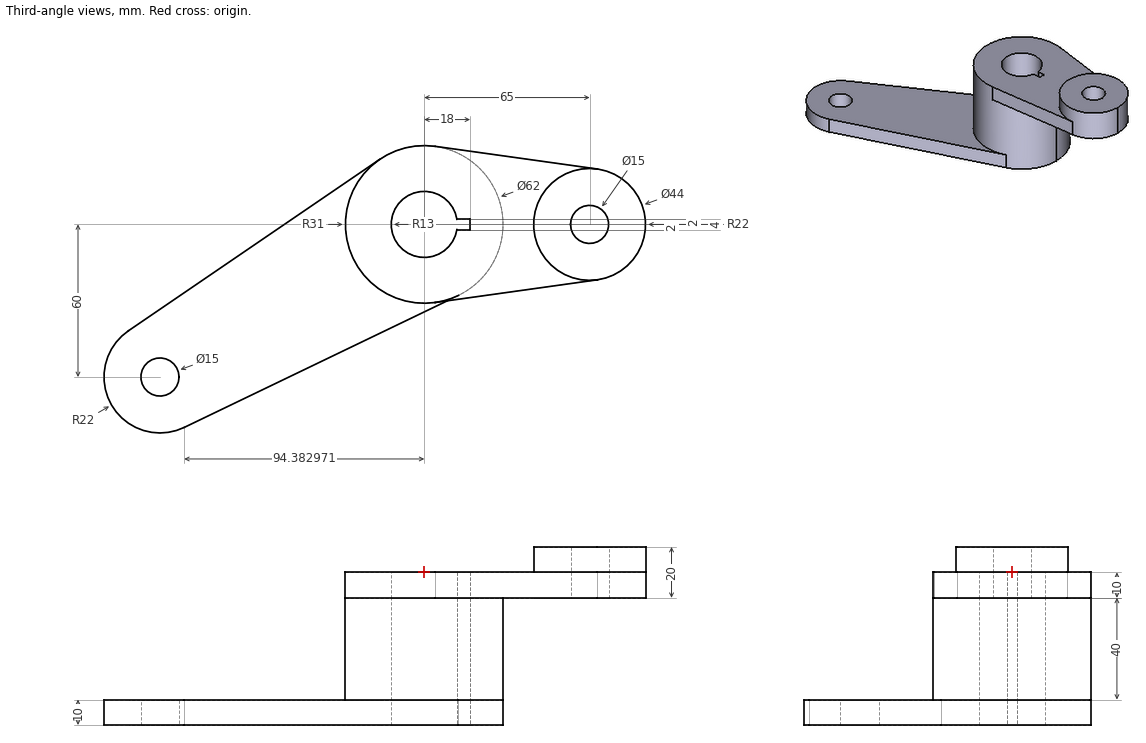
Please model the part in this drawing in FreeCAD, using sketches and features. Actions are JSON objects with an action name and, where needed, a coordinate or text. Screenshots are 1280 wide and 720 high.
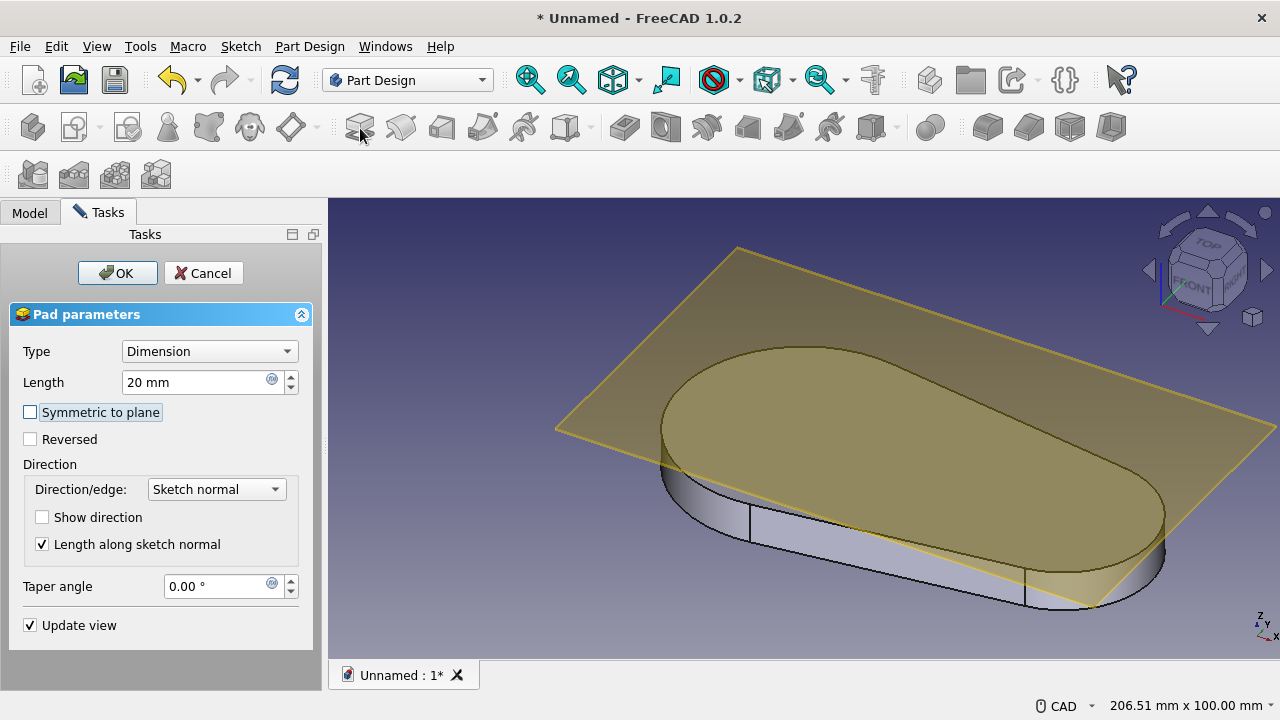
{"action": "left_click", "coordinate": [31, 439]}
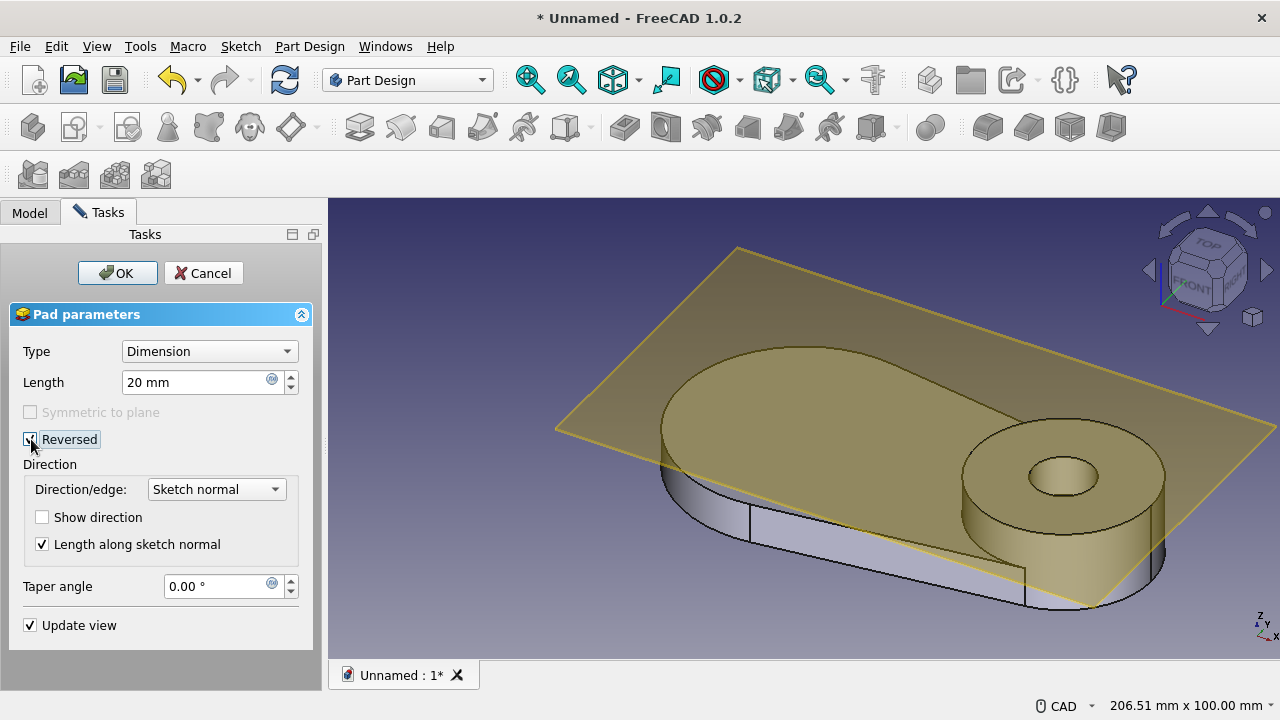
{"action": "left_click", "coordinate": [118, 273]}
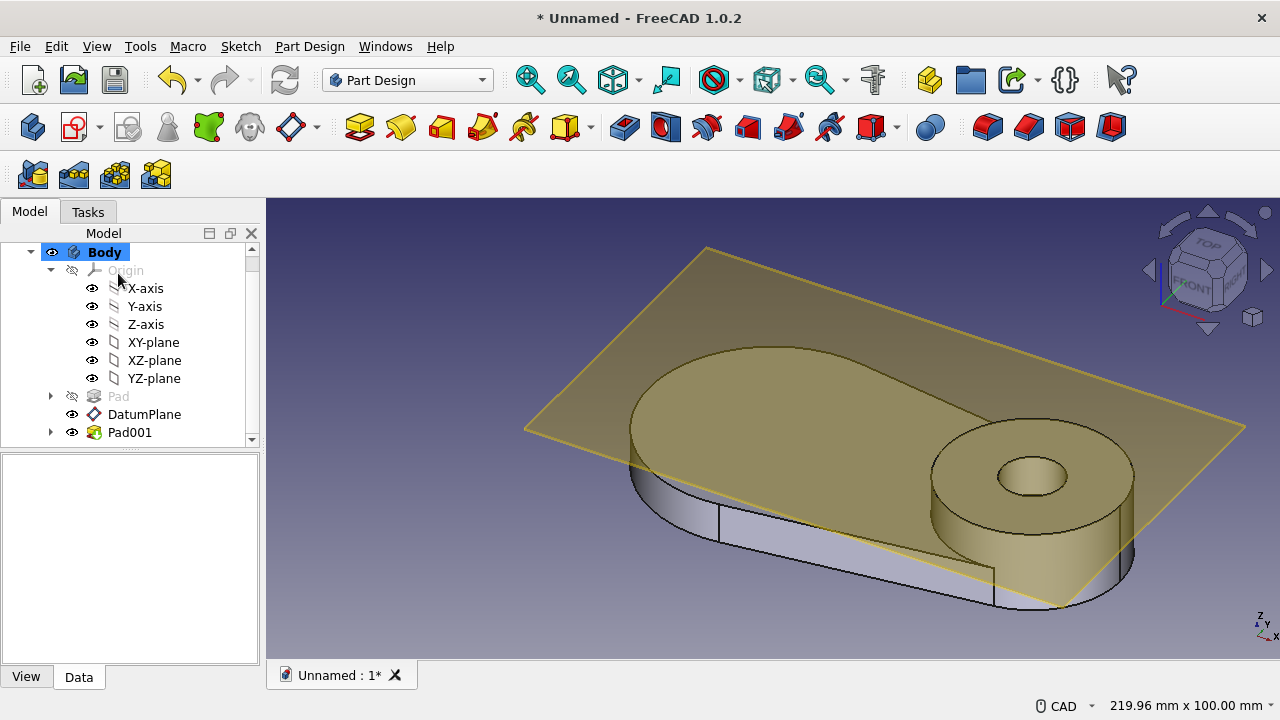
{"action": "left_click", "coordinate": [117, 414]}
{"action": "key", "text": "space"}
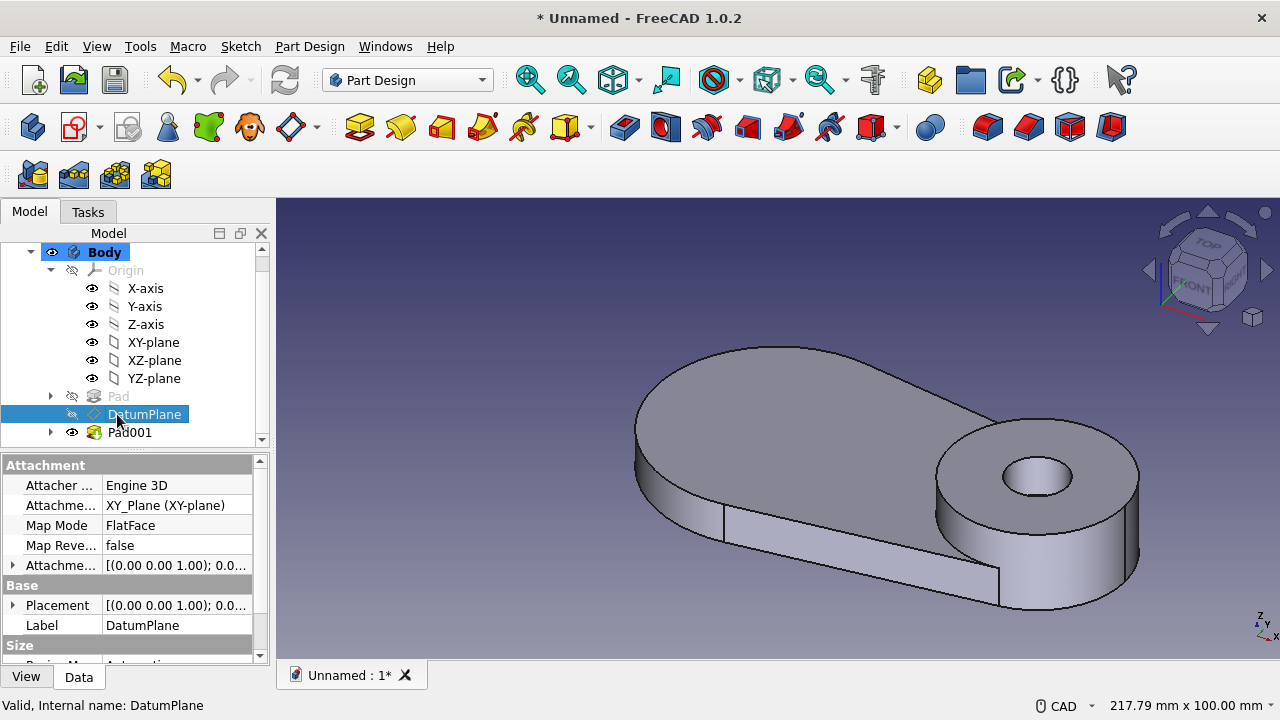
{"action": "key", "text": "5"}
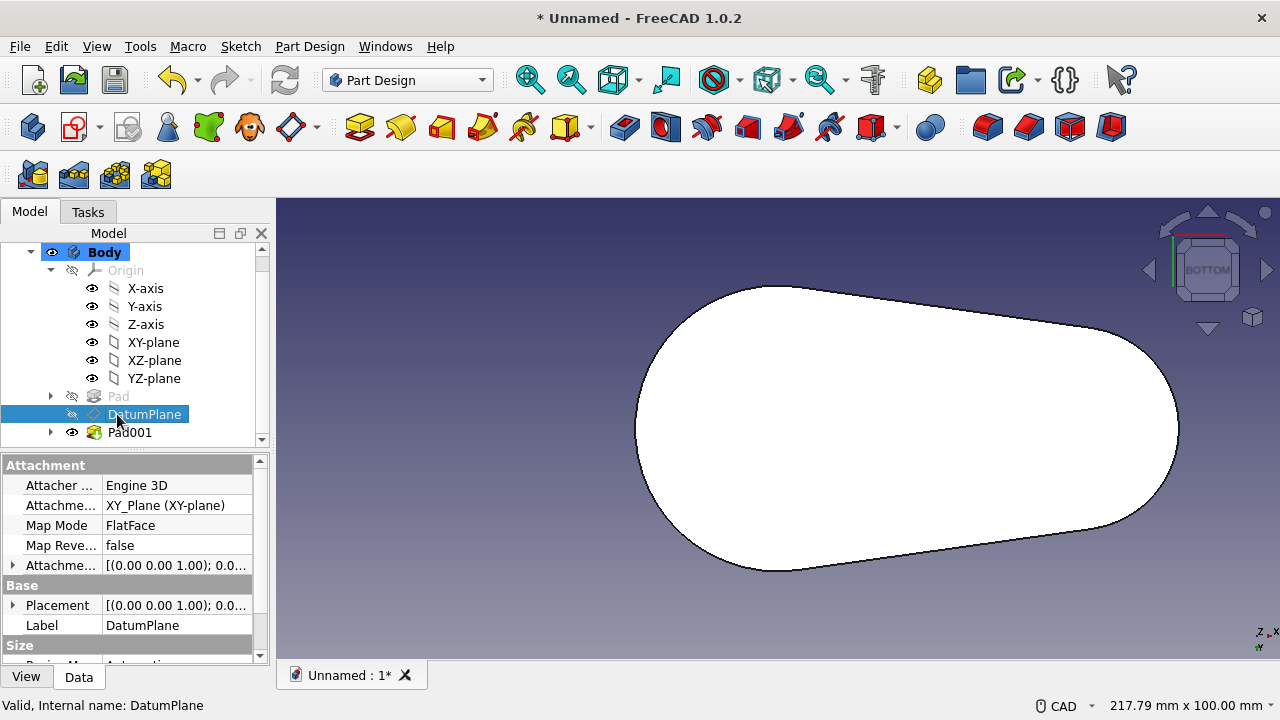
{"action": "left_click", "coordinate": [829, 427]}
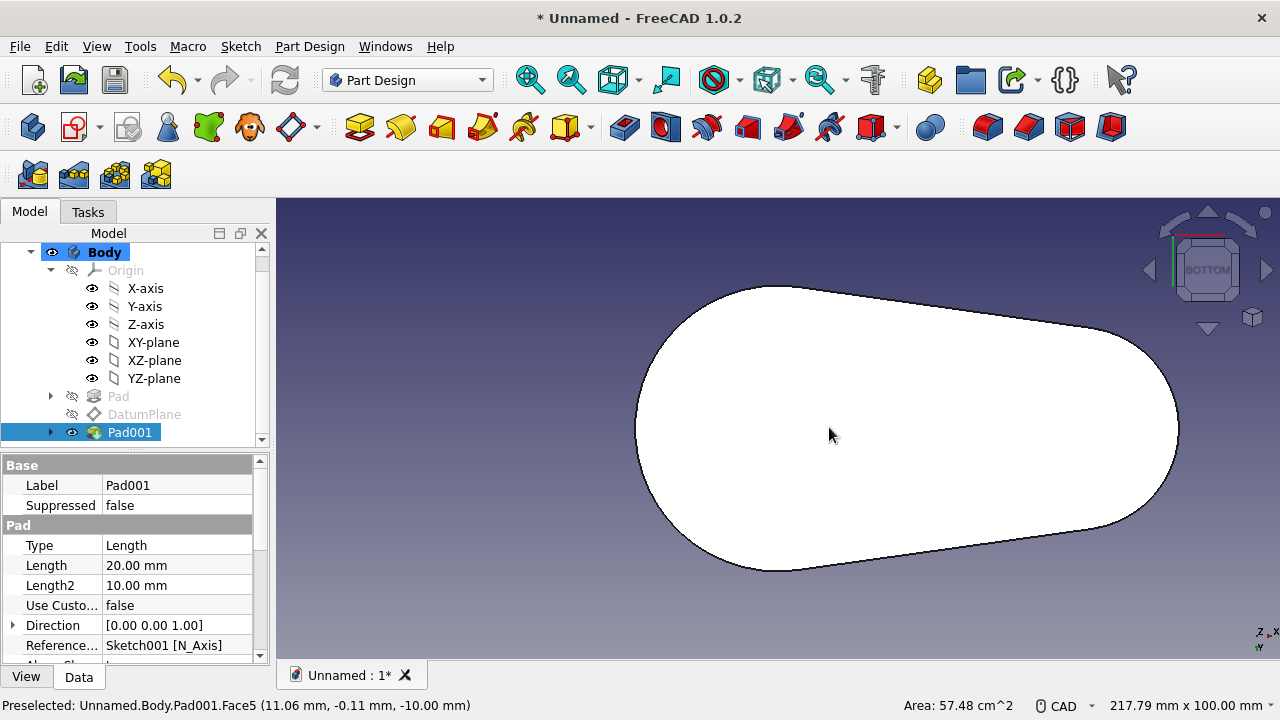
{"action": "left_click", "coordinate": [74, 128]}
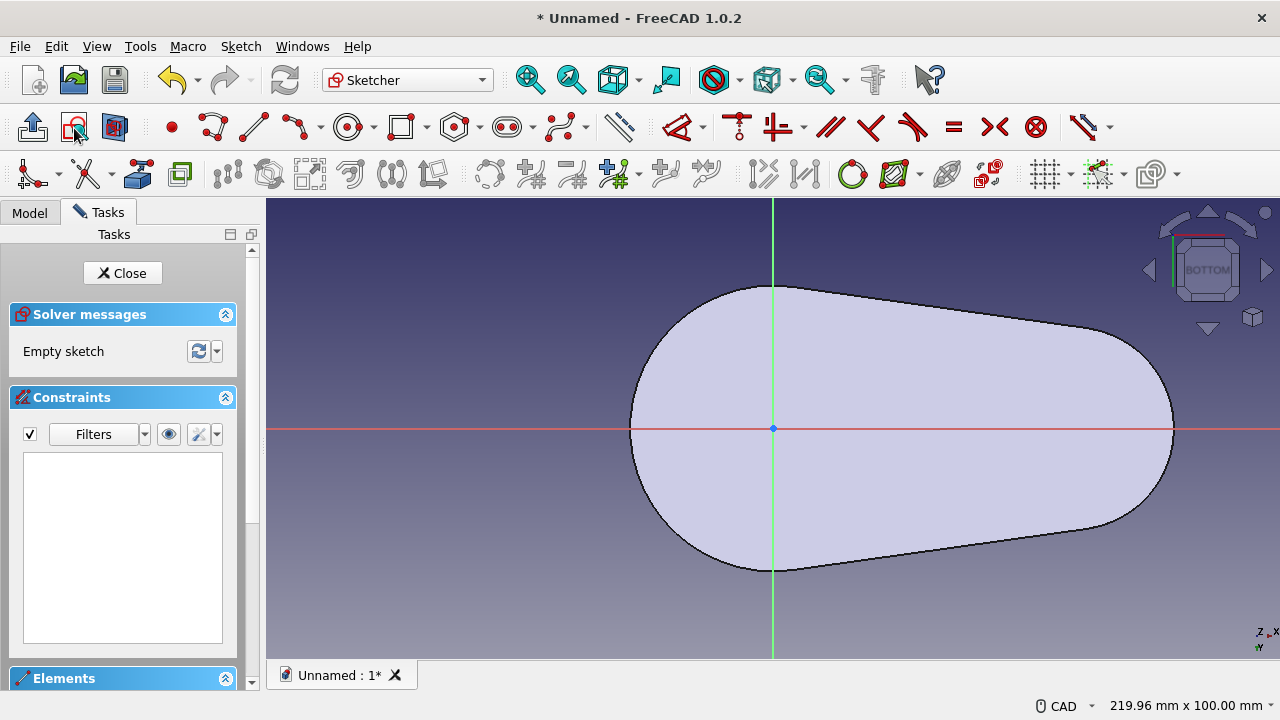
{"action": "scroll", "coordinate": [1115, 429], "scroll_direction": "up", "scroll_amount": 7}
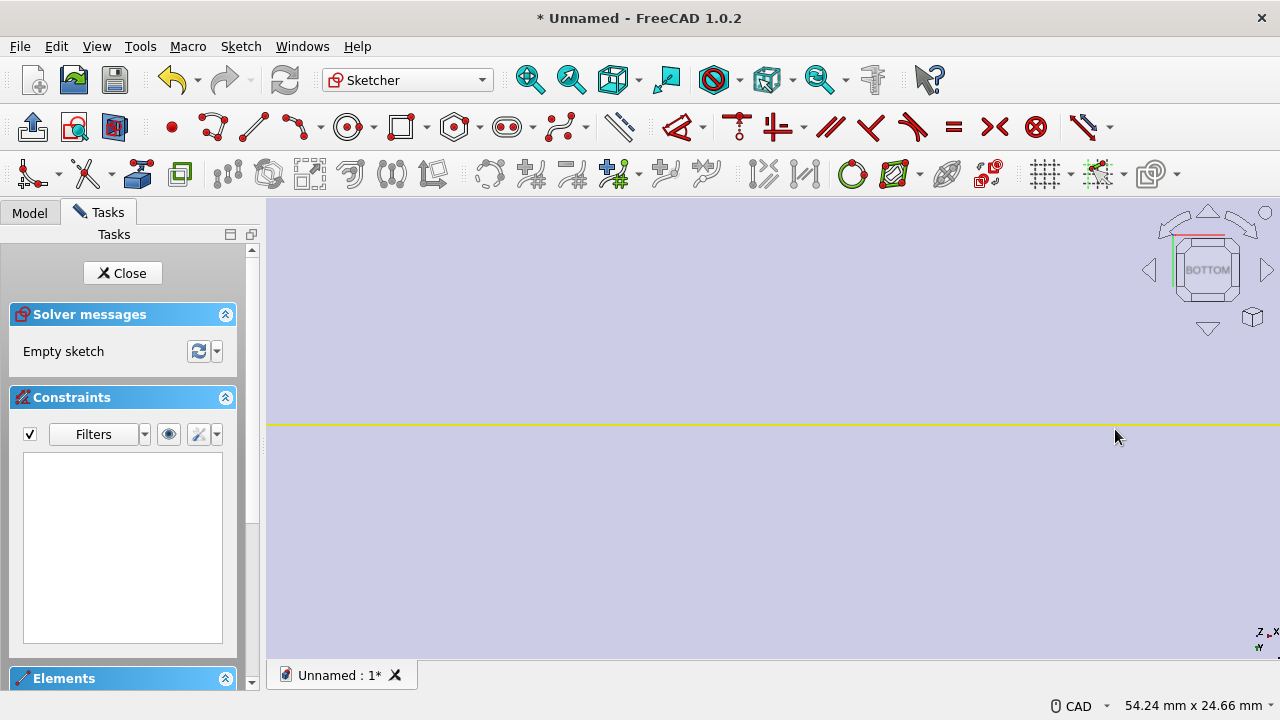
{"action": "key", "text": "g c"}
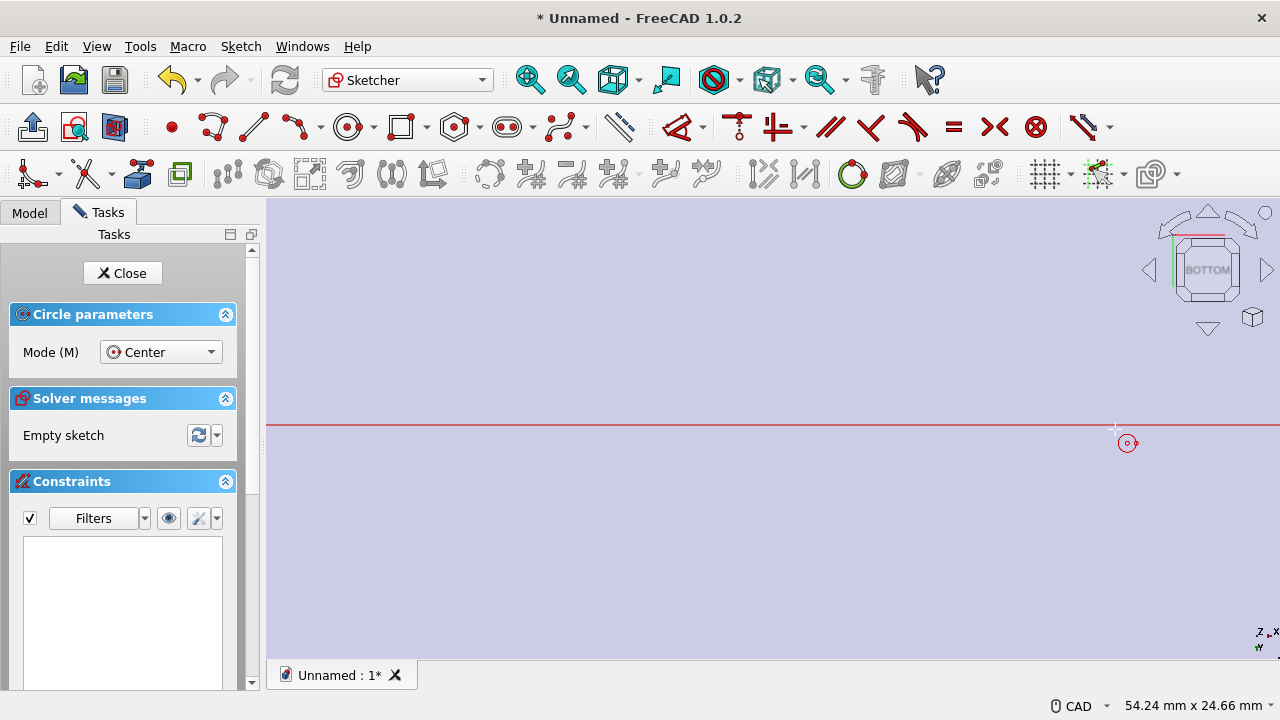
{"action": "left_click", "coordinate": [941, 425]}
{"action": "left_click", "coordinate": [1040, 326]}
{"action": "key", "text": "Escape"}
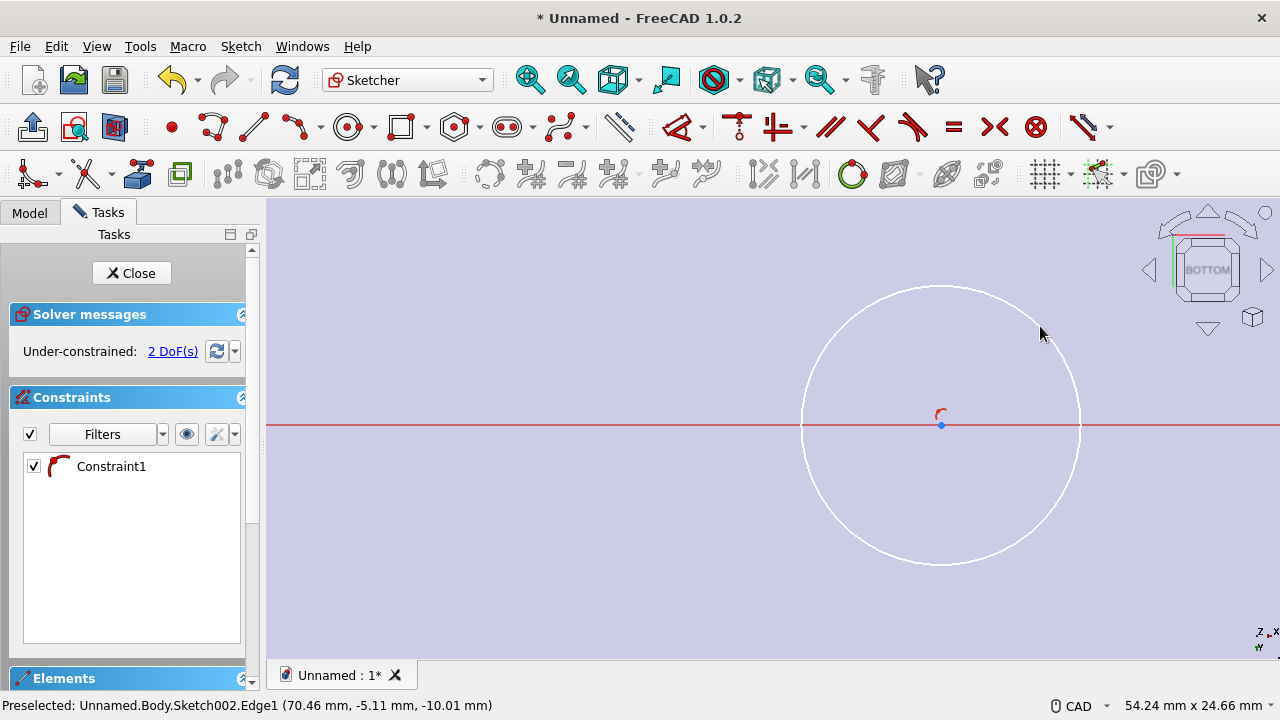
{"action": "key", "text": "d"}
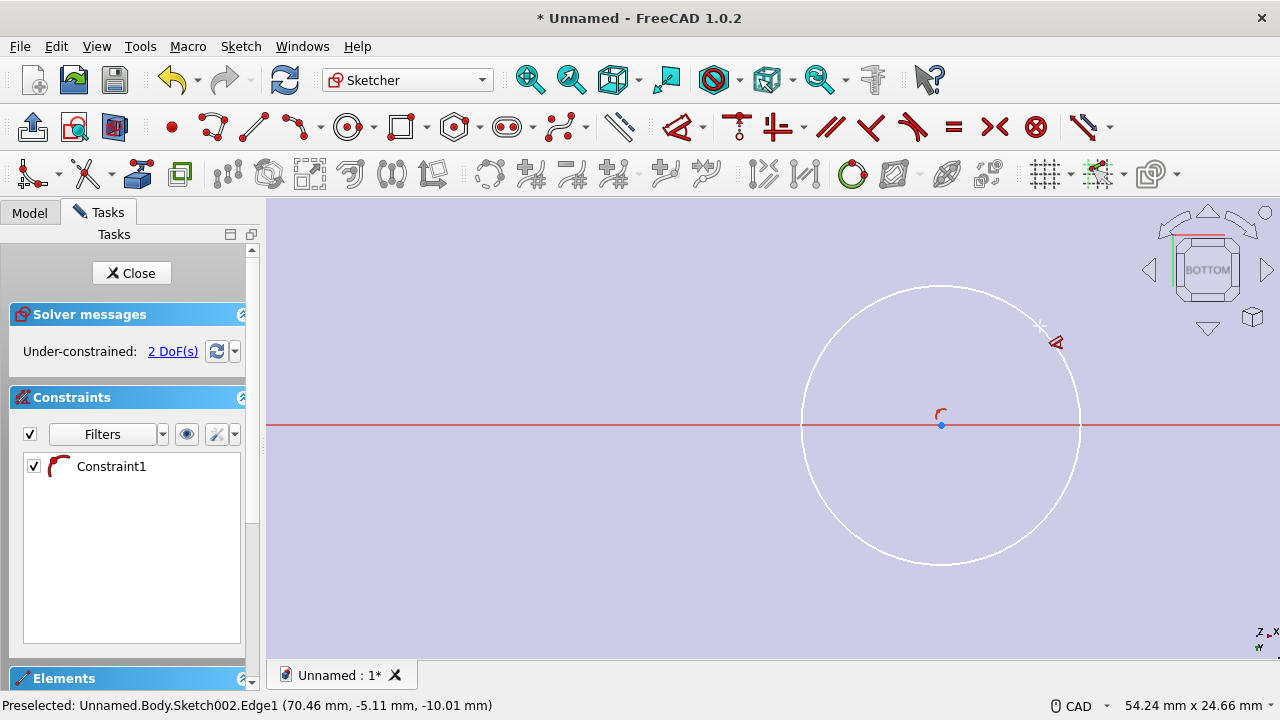
{"action": "left_click", "coordinate": [1039, 326]}
{"action": "left_click", "coordinate": [1061, 303]}